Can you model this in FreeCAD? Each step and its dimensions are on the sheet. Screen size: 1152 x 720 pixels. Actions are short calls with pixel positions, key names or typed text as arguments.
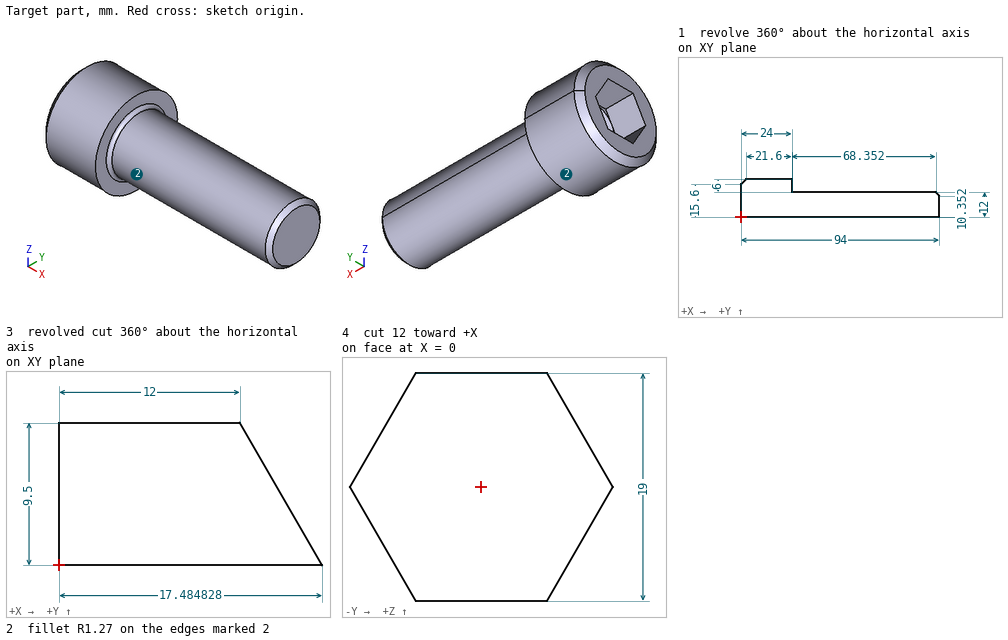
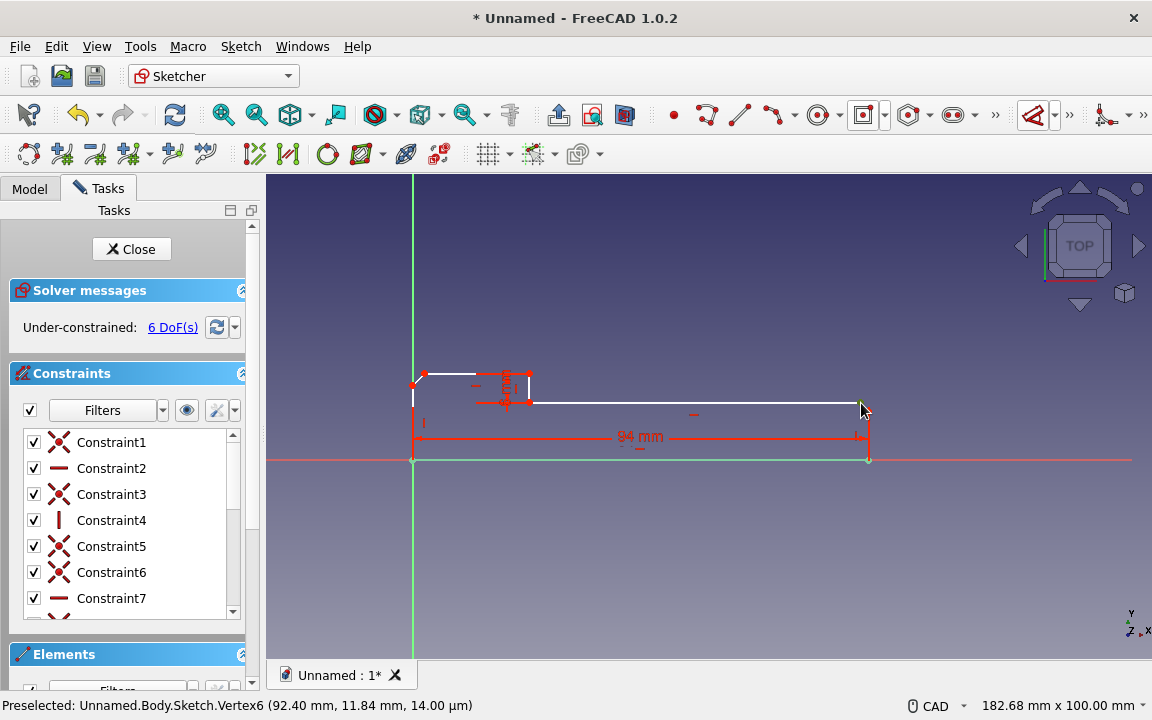
key(i)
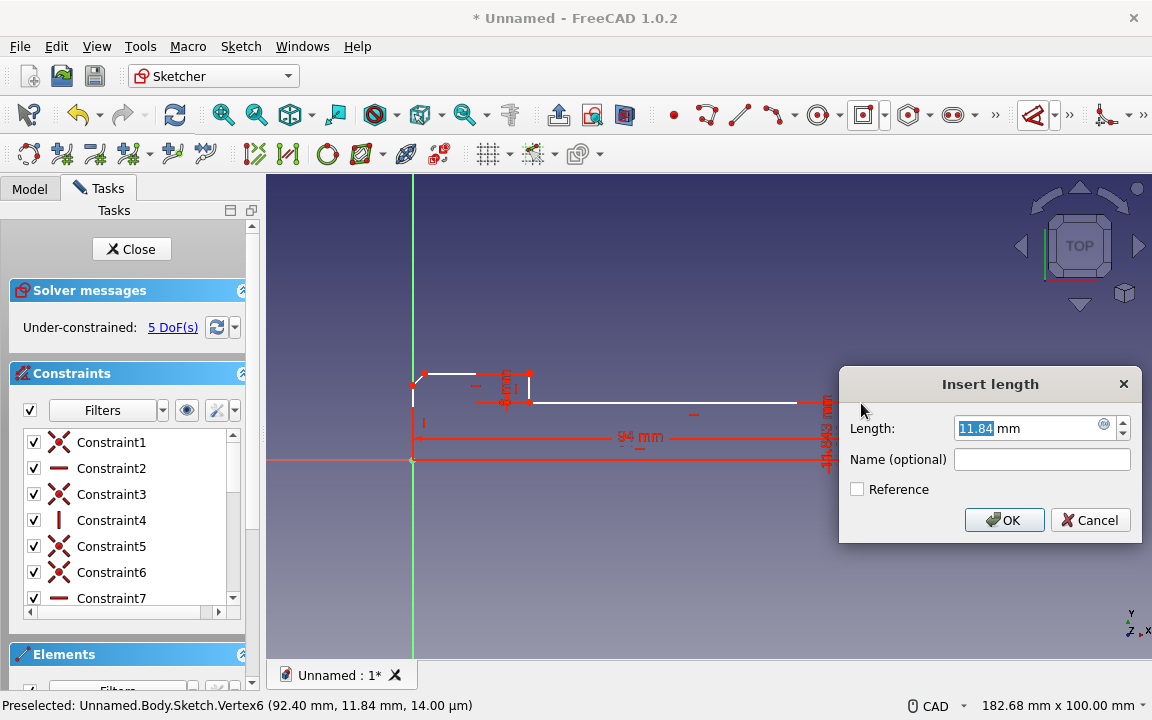
text(12)
key(Return)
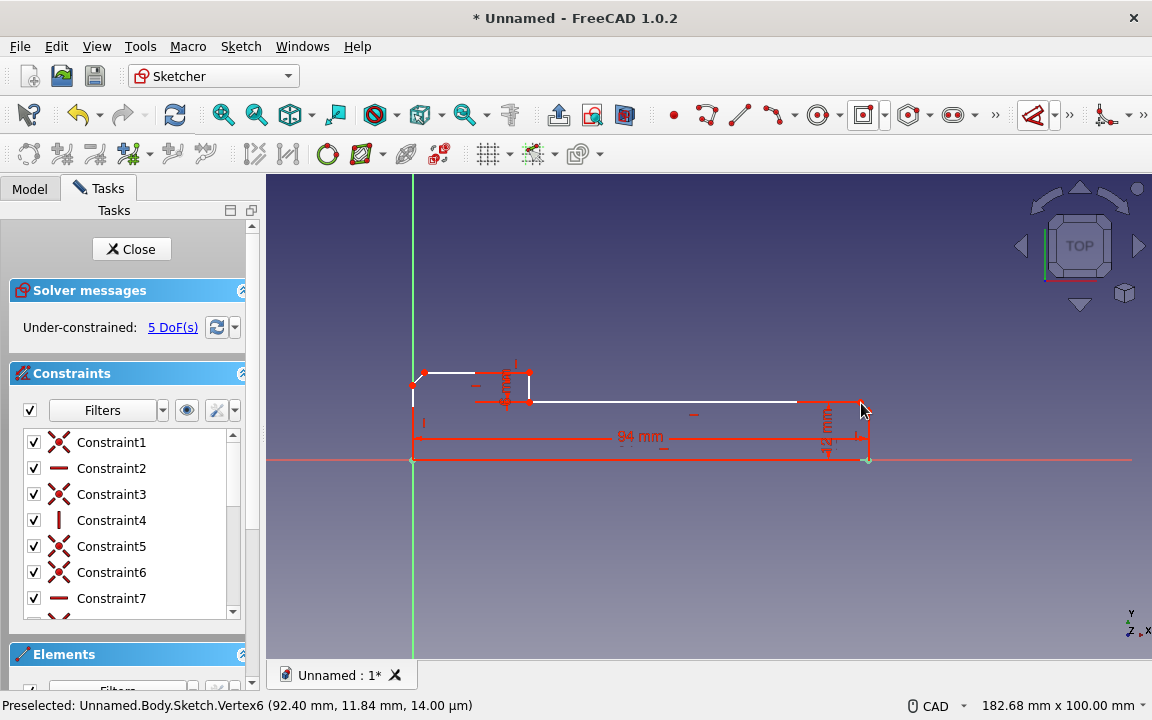
click(529, 402)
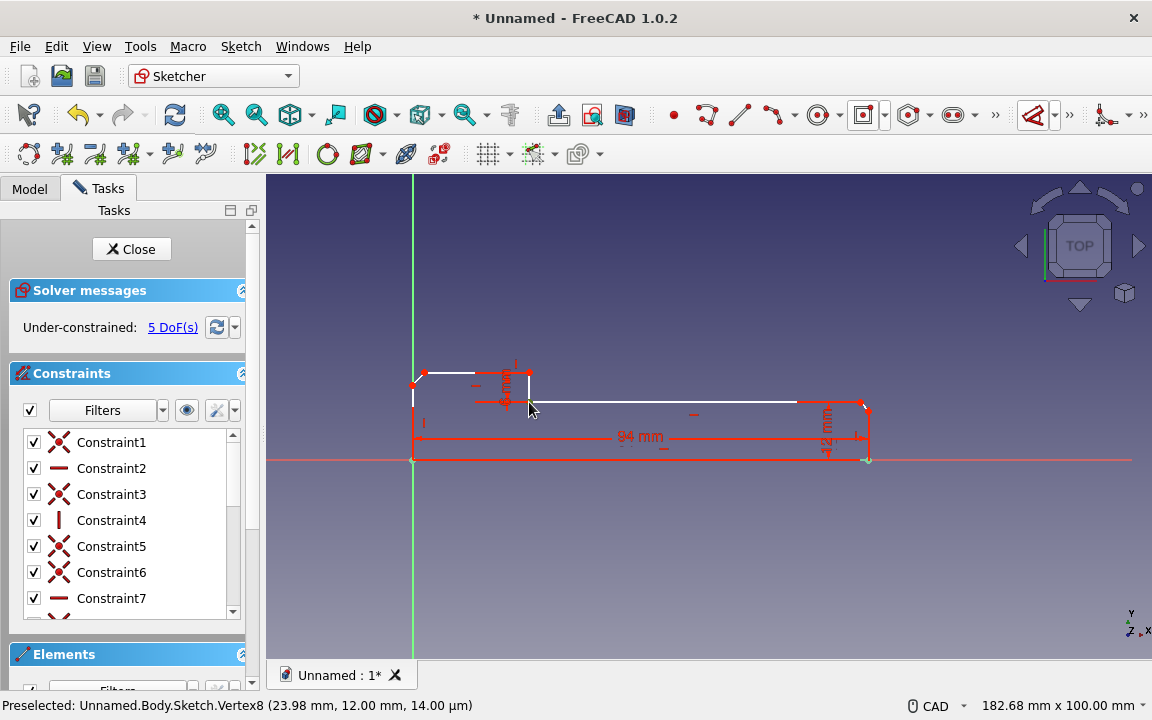
click(1054, 116)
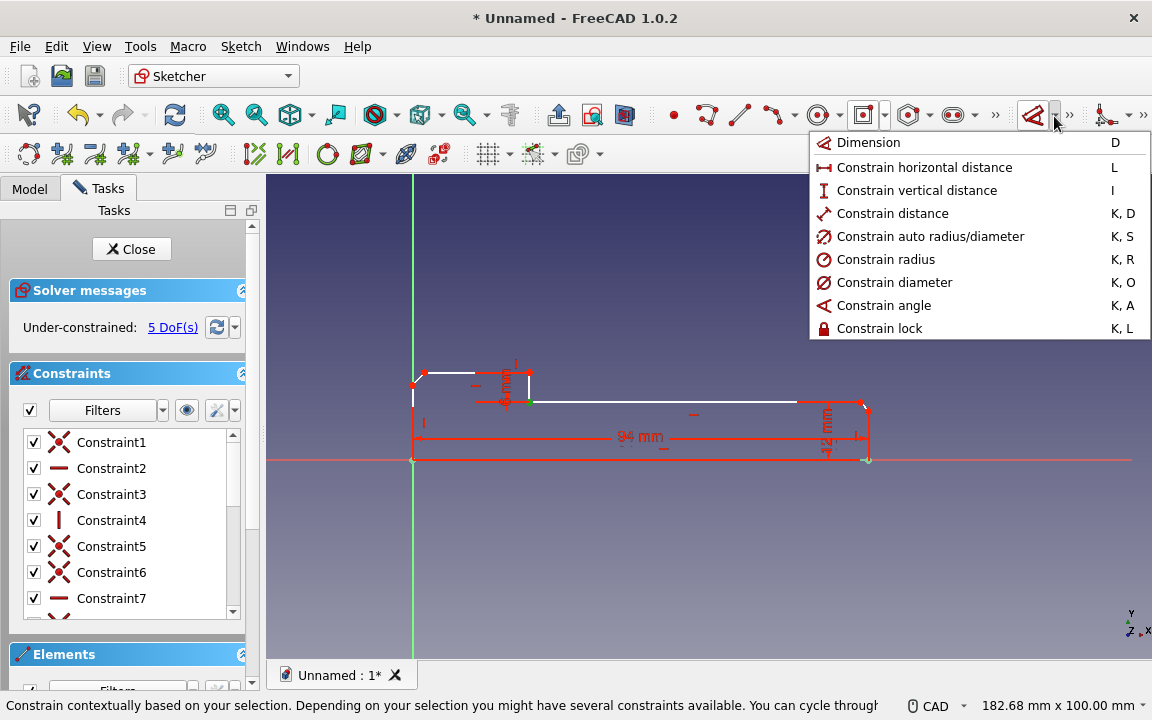
click(980, 168)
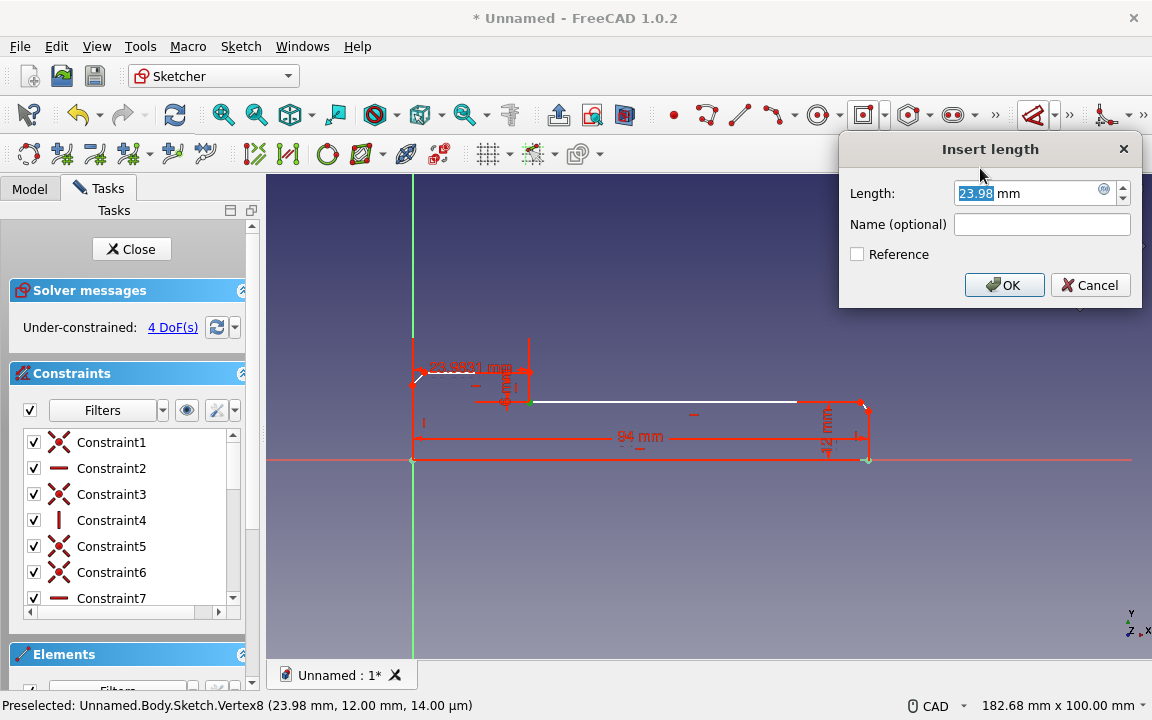
text(24)
key(Return)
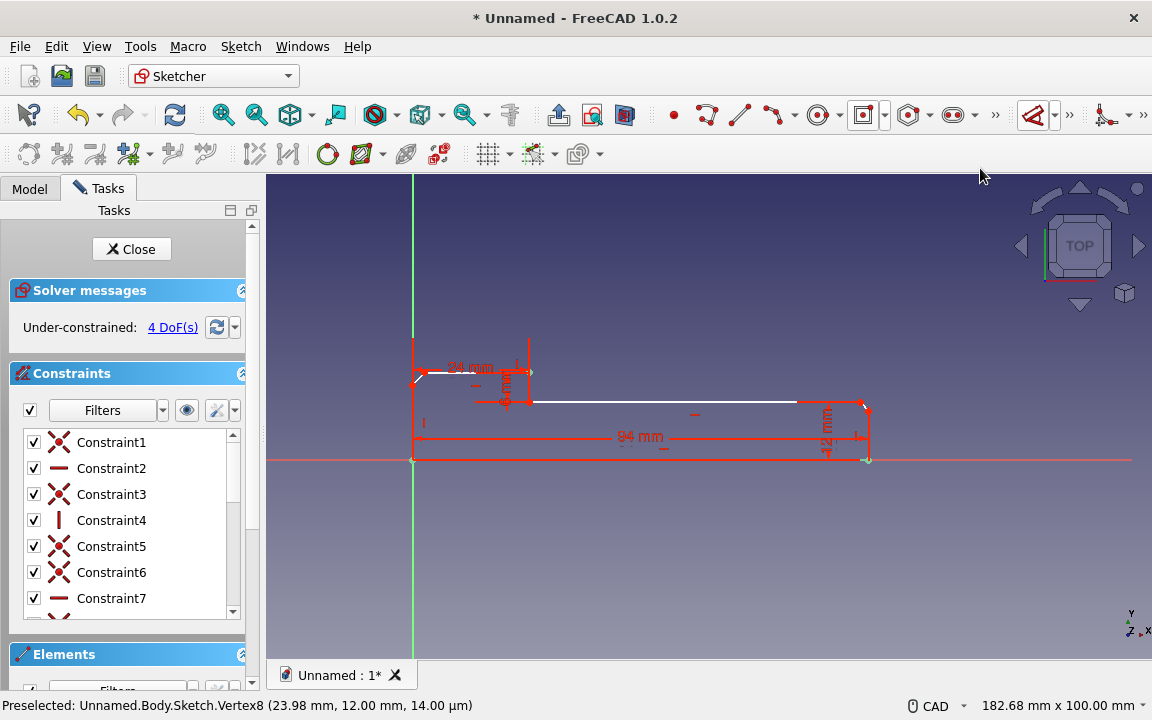
click(498, 373)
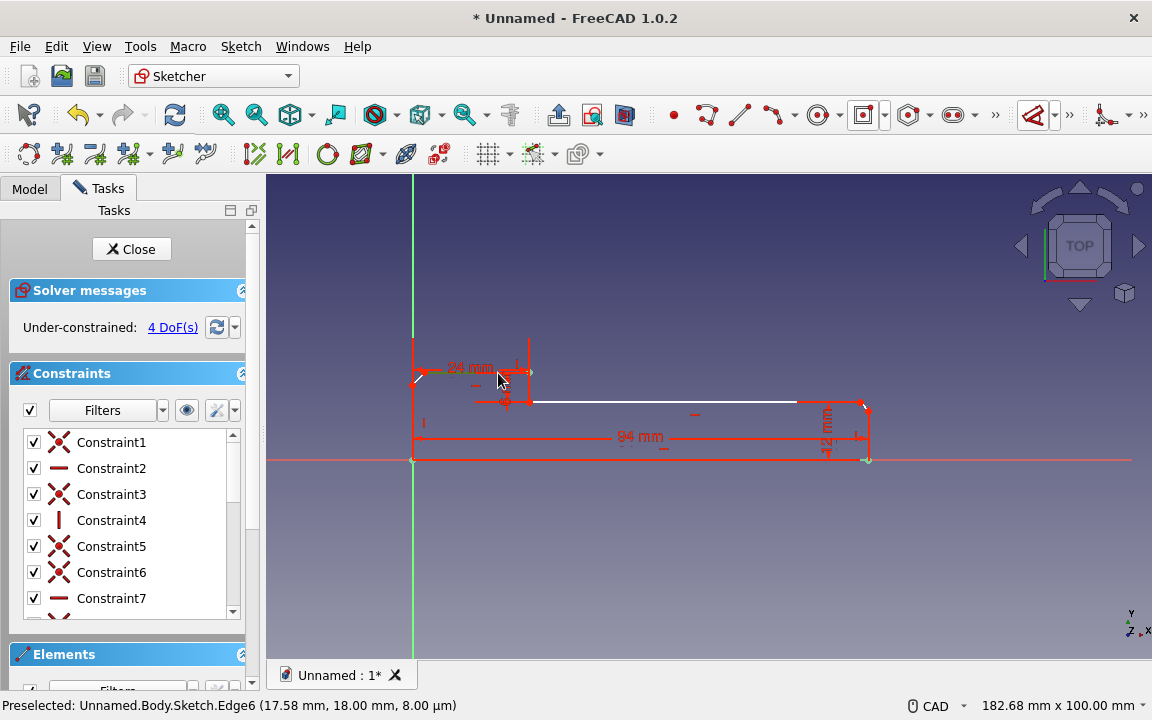
click(1054, 116)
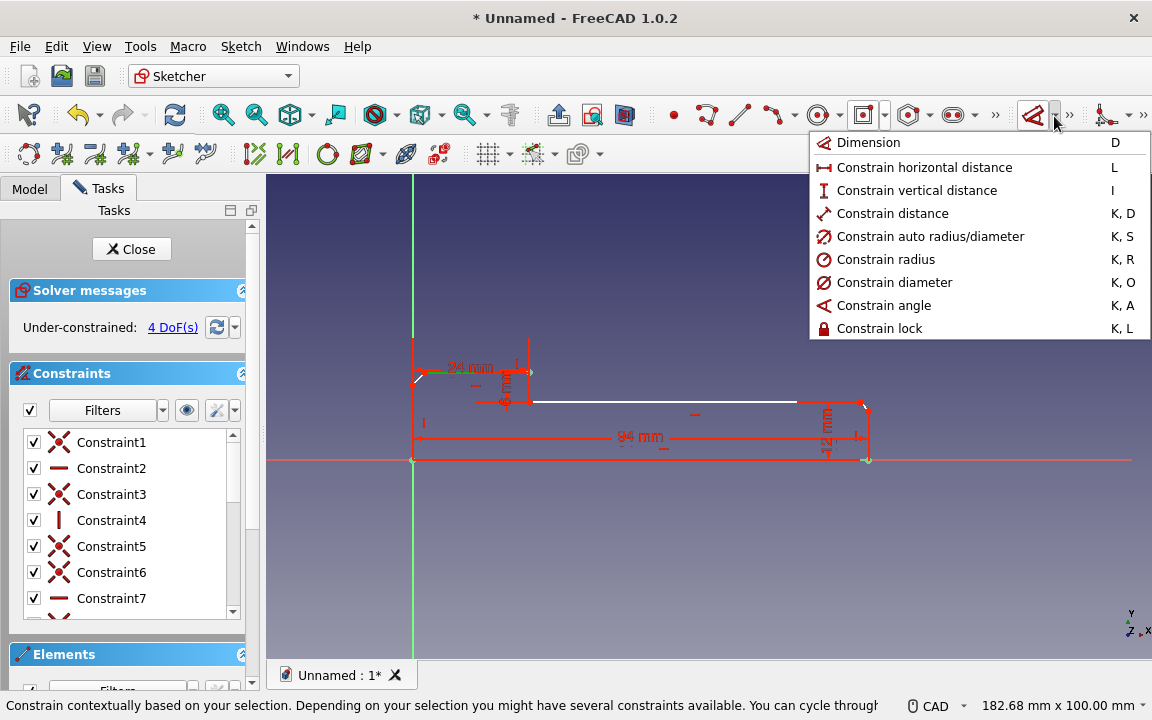
click(980, 168)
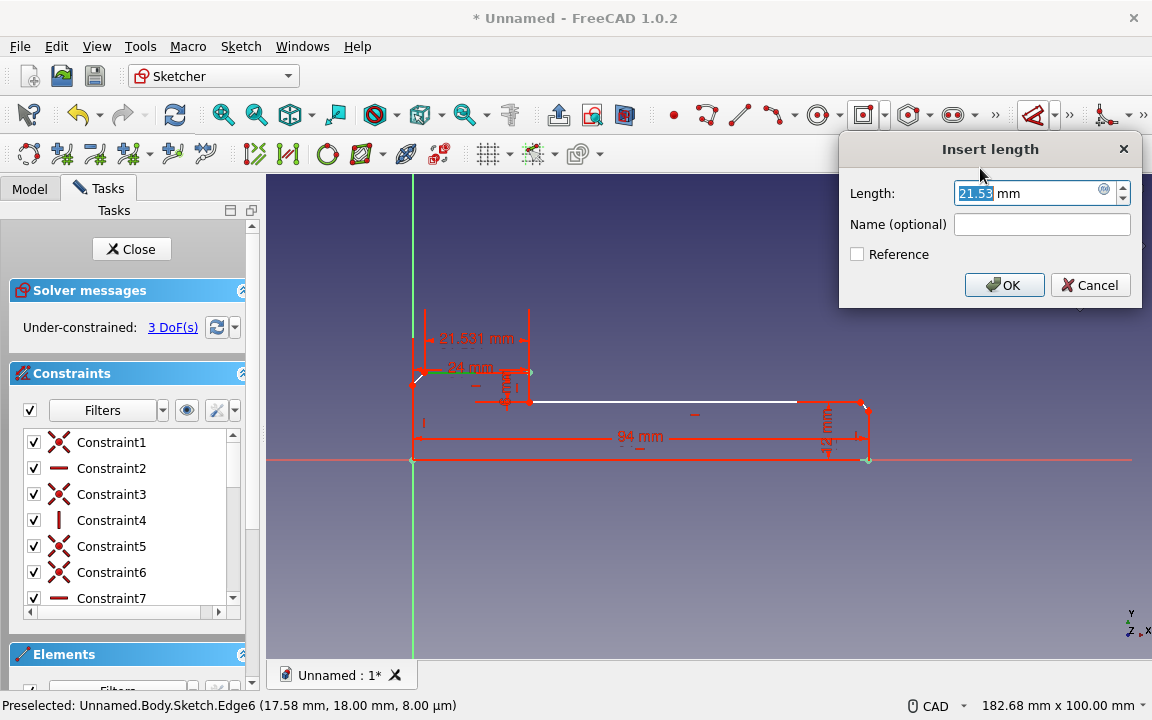
text(21.6)
key(Return)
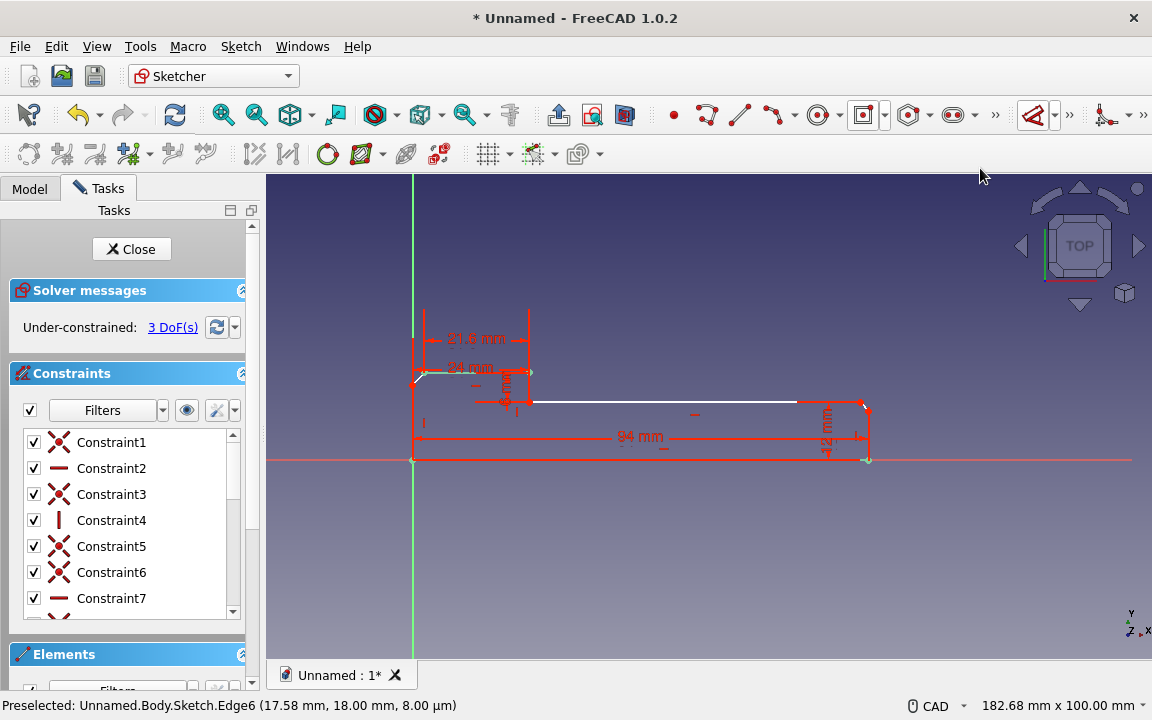
click(413, 408)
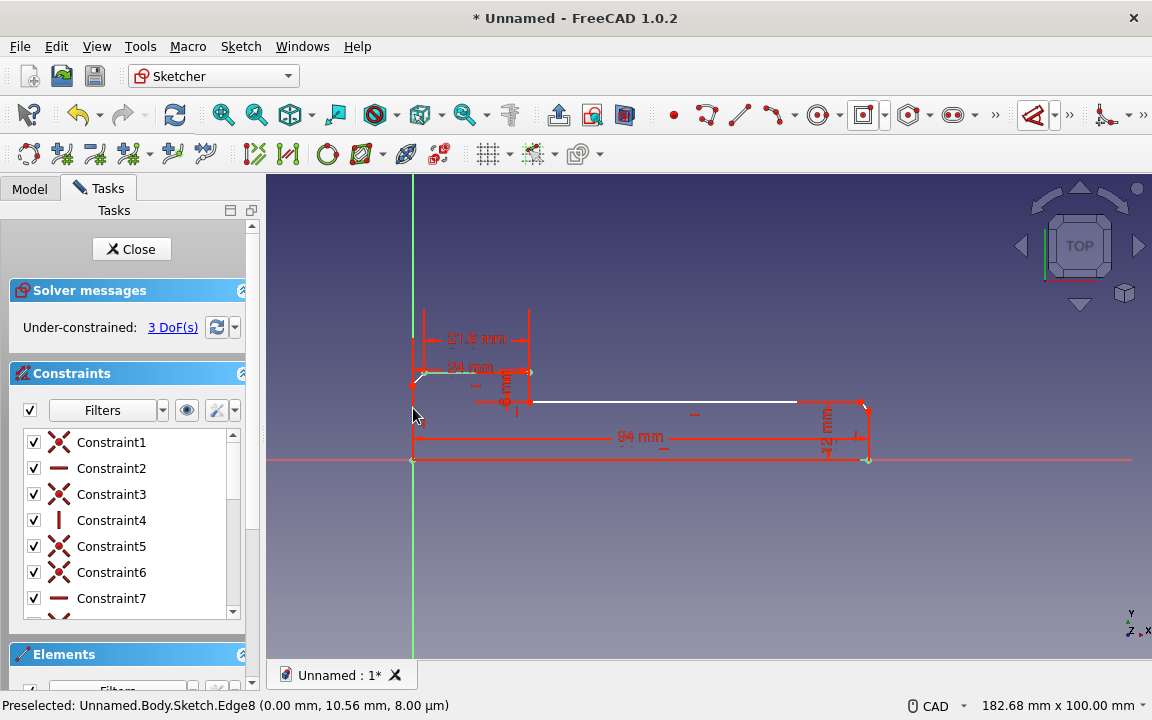
key(i)